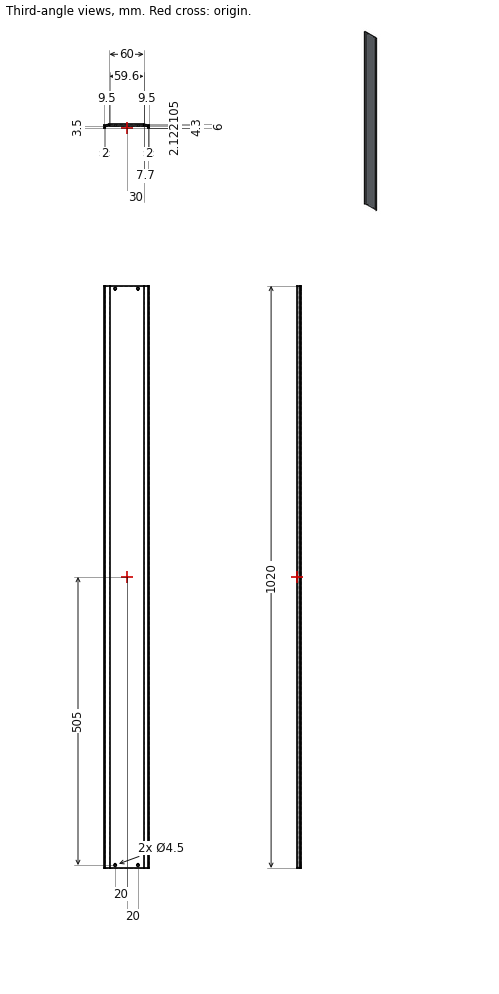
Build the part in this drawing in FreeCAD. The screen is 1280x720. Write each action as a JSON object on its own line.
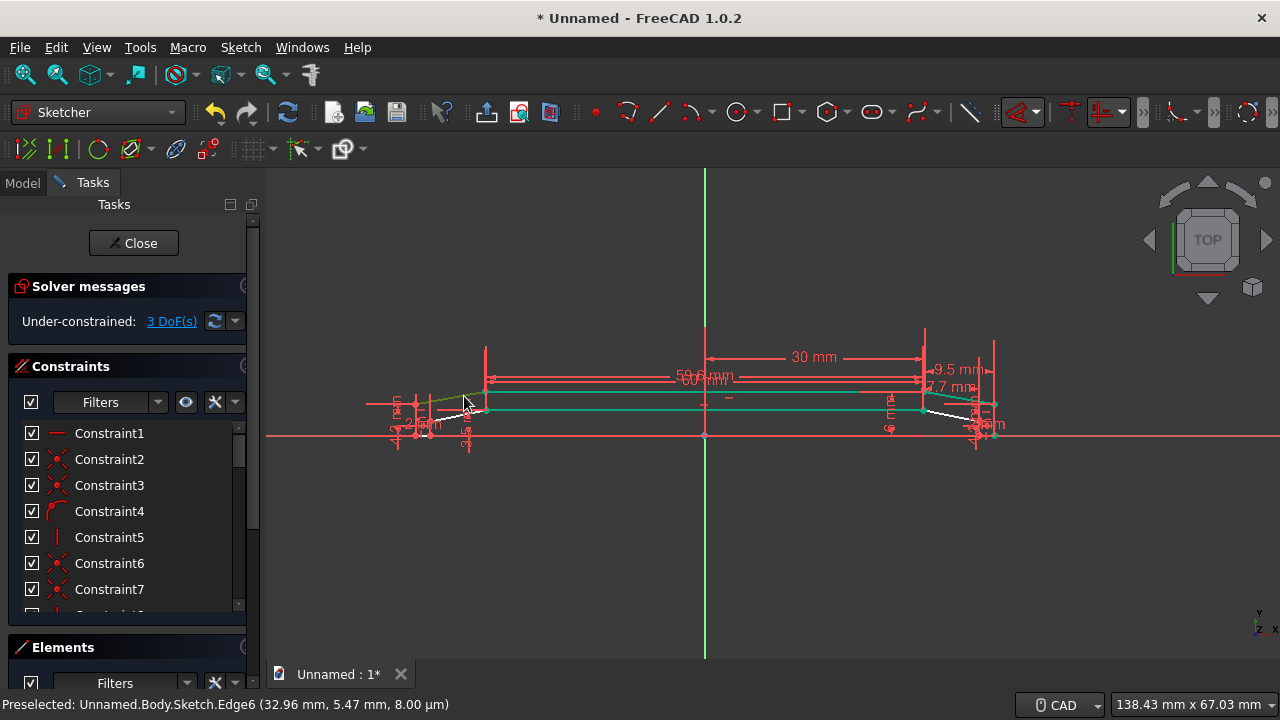
{"action": "key", "text": "l"}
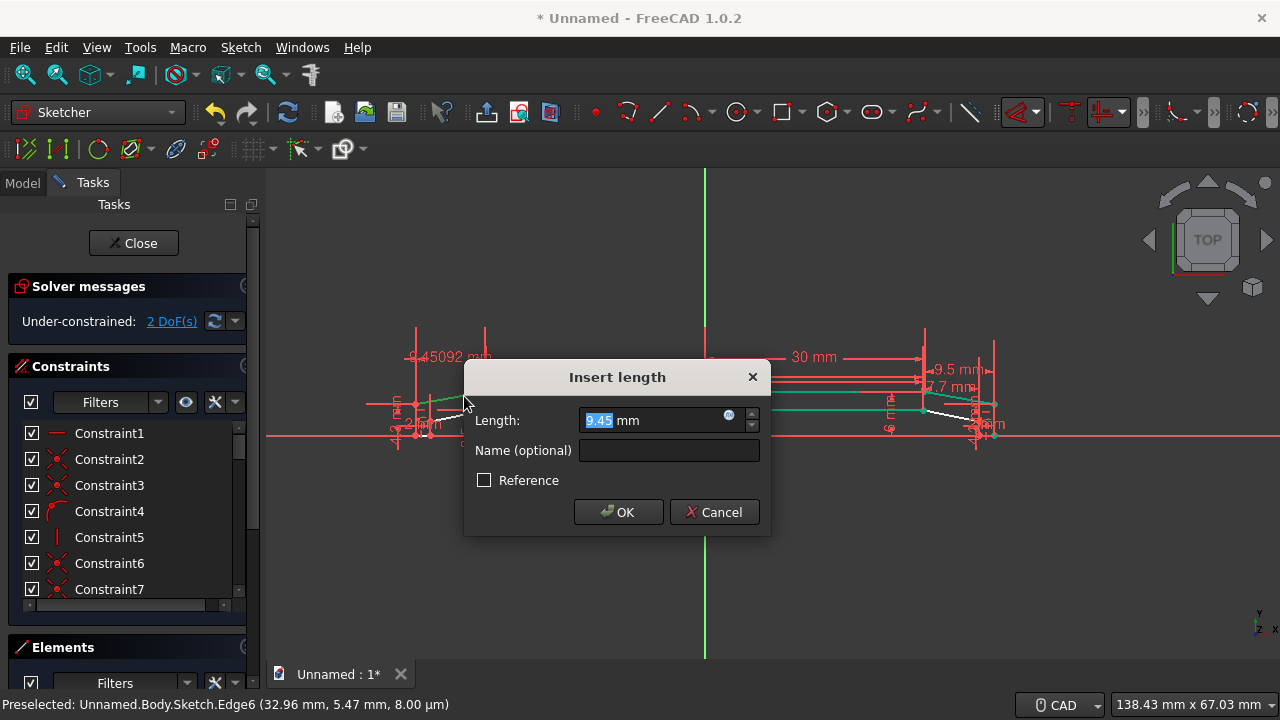
{"action": "type", "text": "9.5"}
{"action": "key", "text": "Return"}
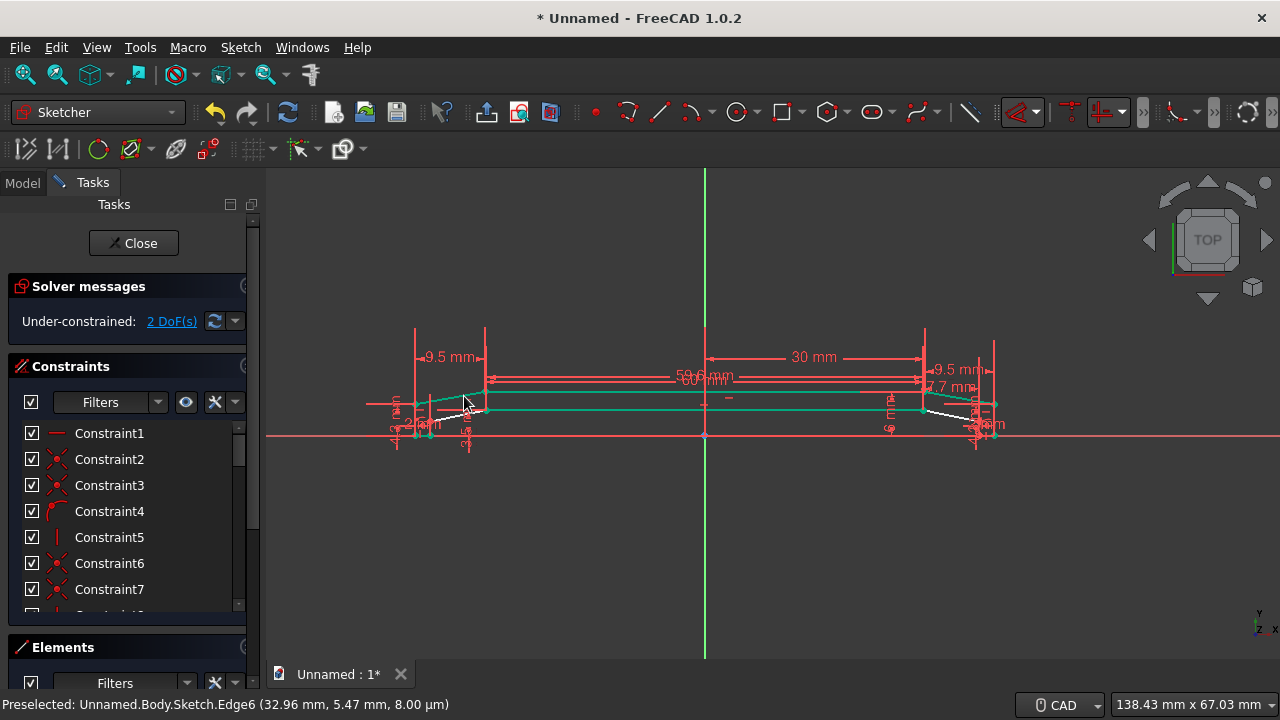
{"action": "scroll", "coordinate": [979, 429], "scroll_direction": "up", "scroll_amount": 5}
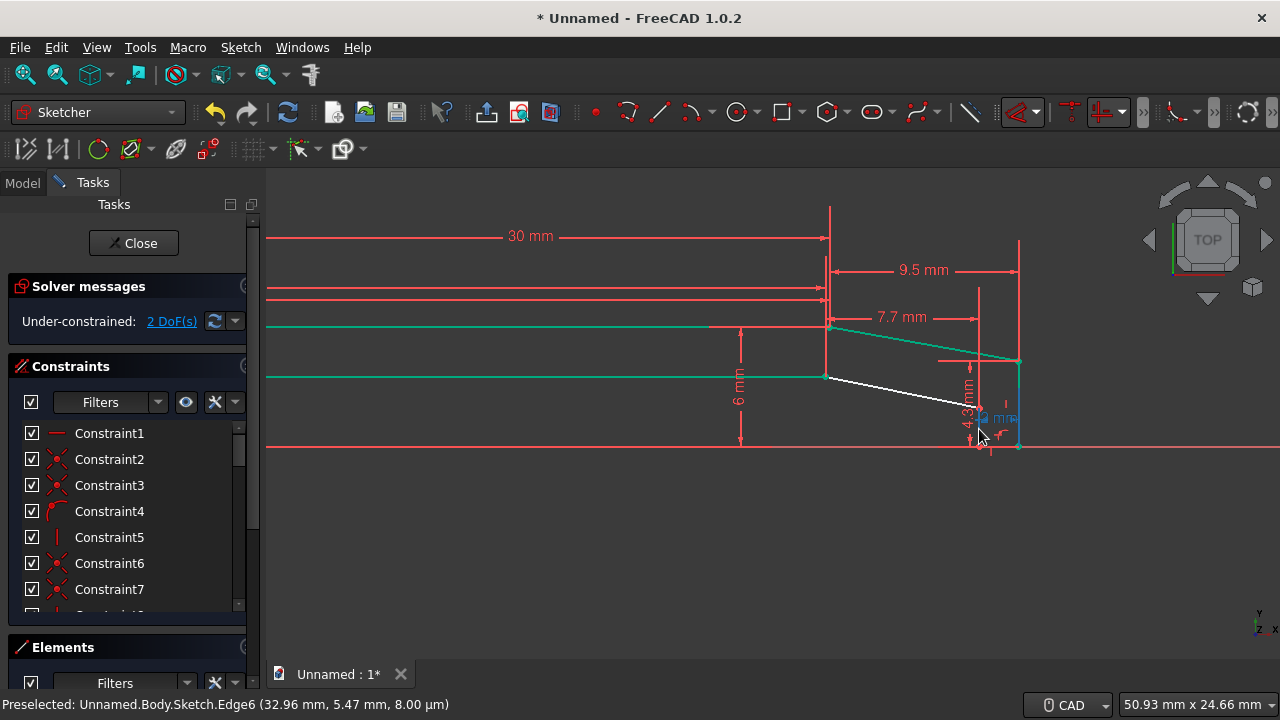
{"action": "left_click", "coordinate": [979, 427]}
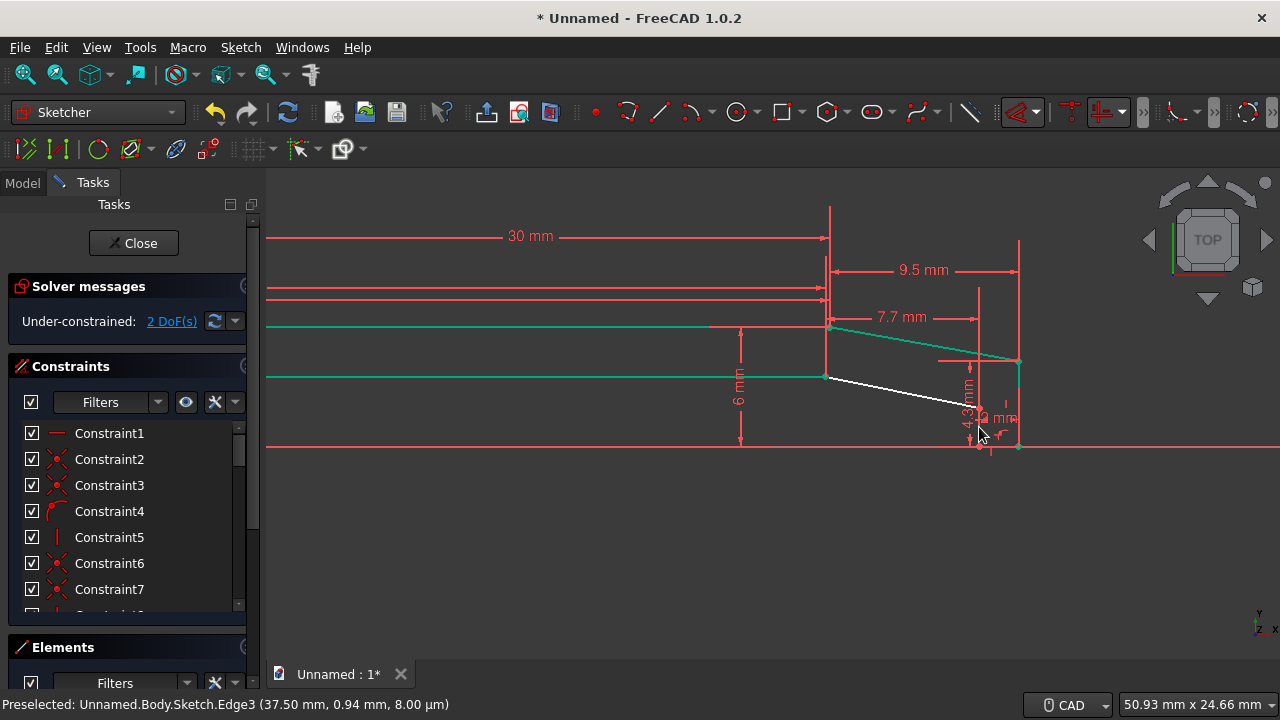
{"action": "key", "text": "i"}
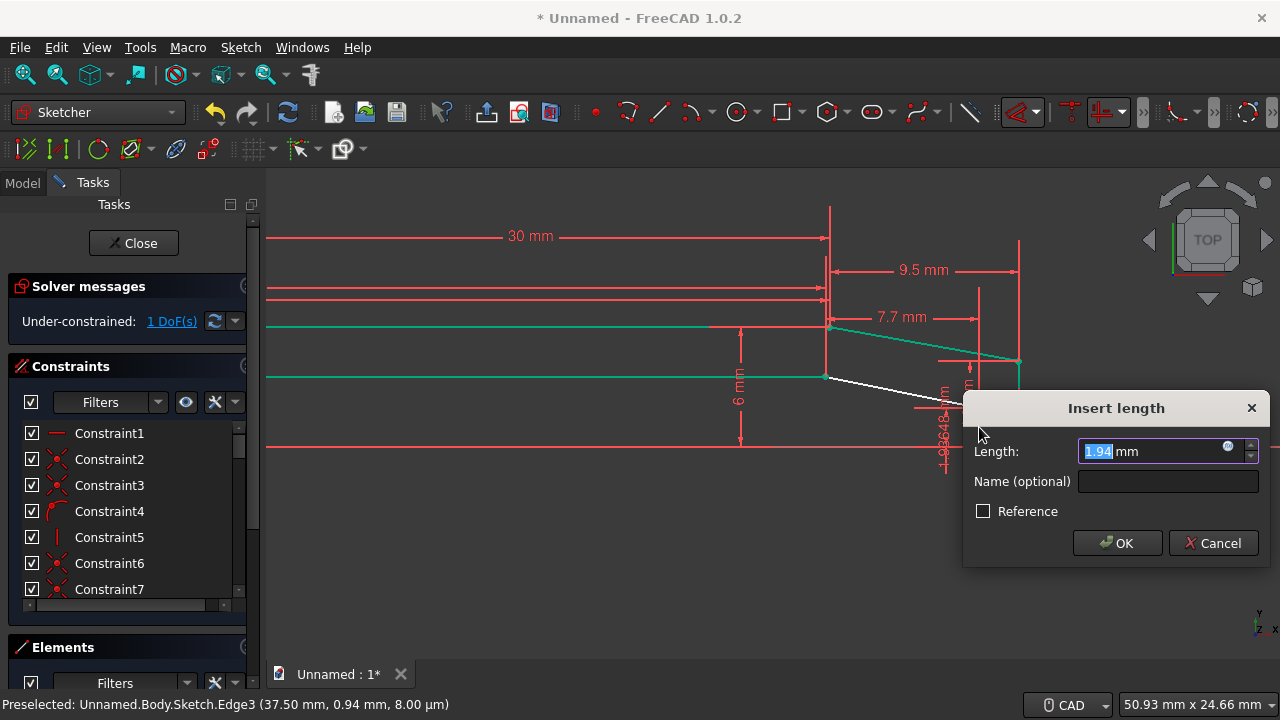
{"action": "type", "text": "2.122105"}
{"action": "key", "text": "Return"}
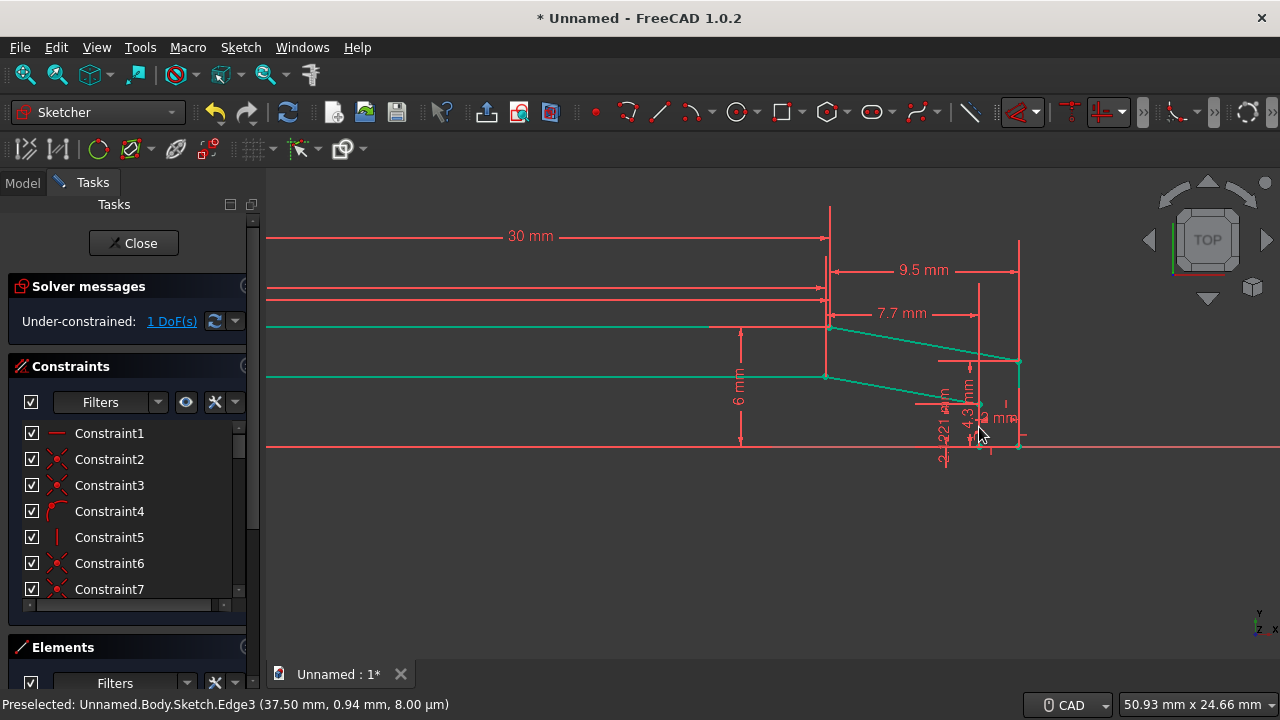
{"action": "scroll", "coordinate": [979, 429], "scroll_direction": "down", "scroll_amount": 5}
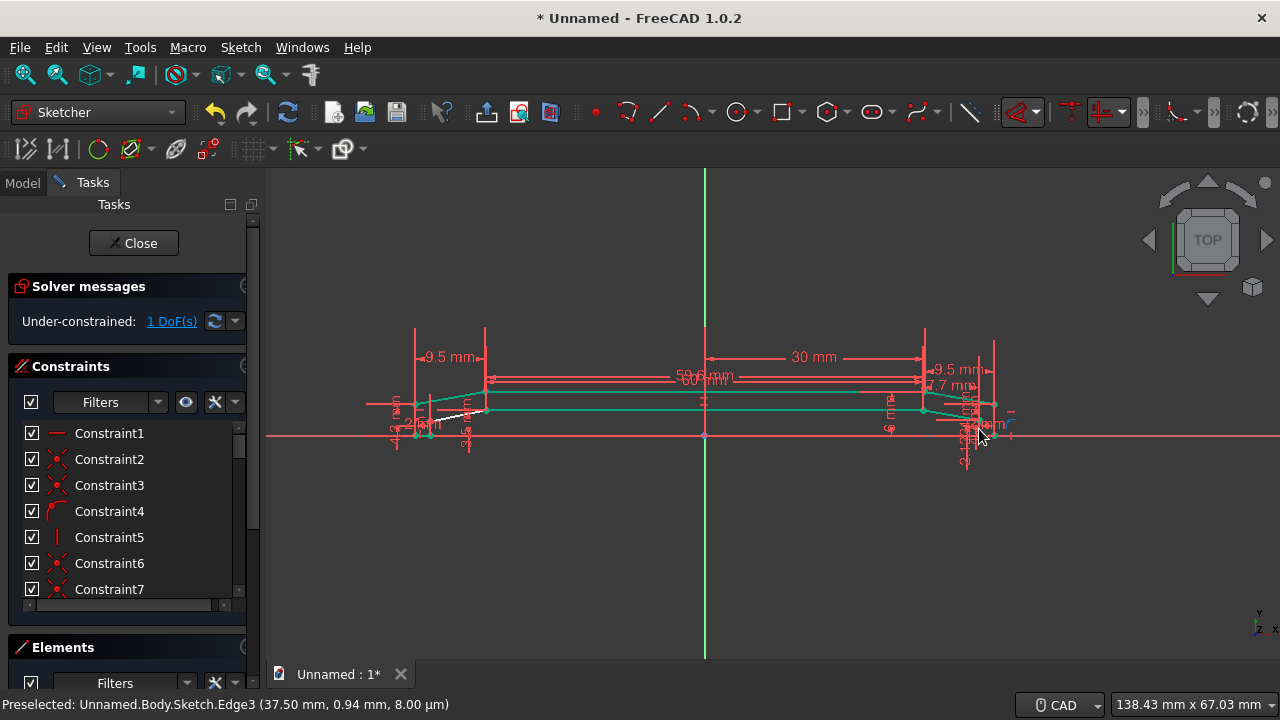
{"action": "scroll", "coordinate": [430, 432], "scroll_direction": "up", "scroll_amount": 6}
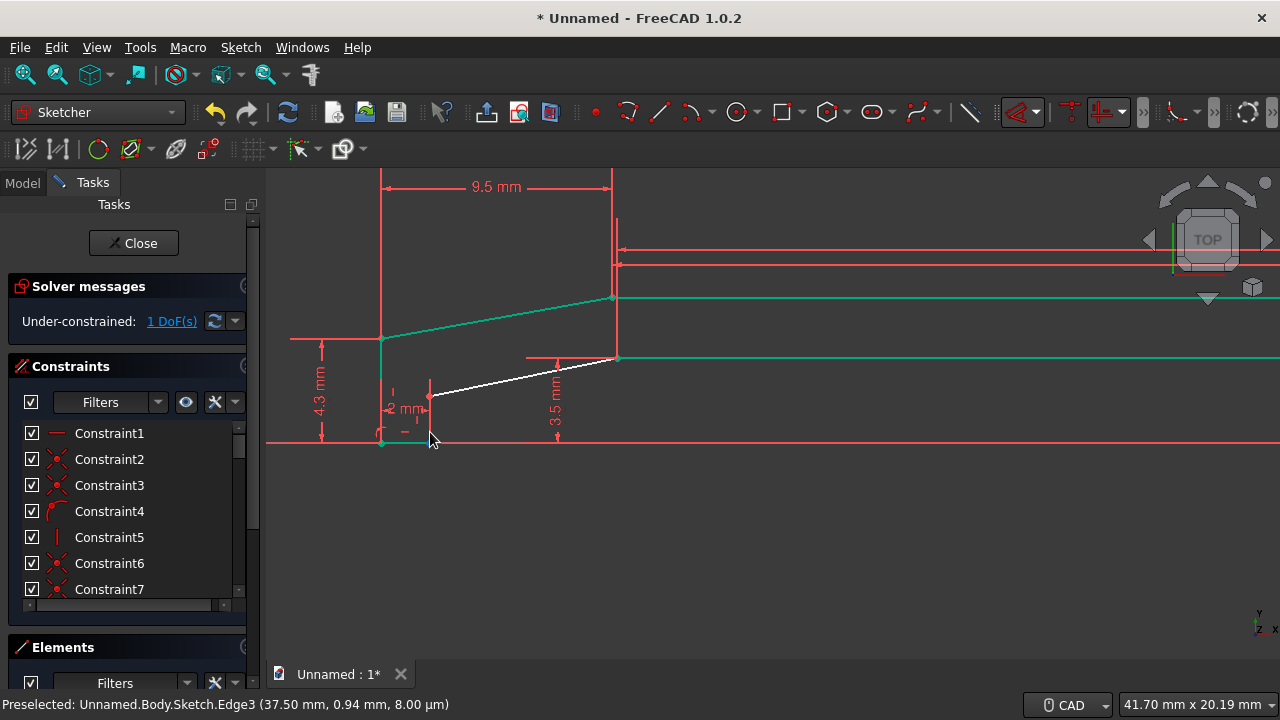
{"action": "left_click", "coordinate": [430, 429]}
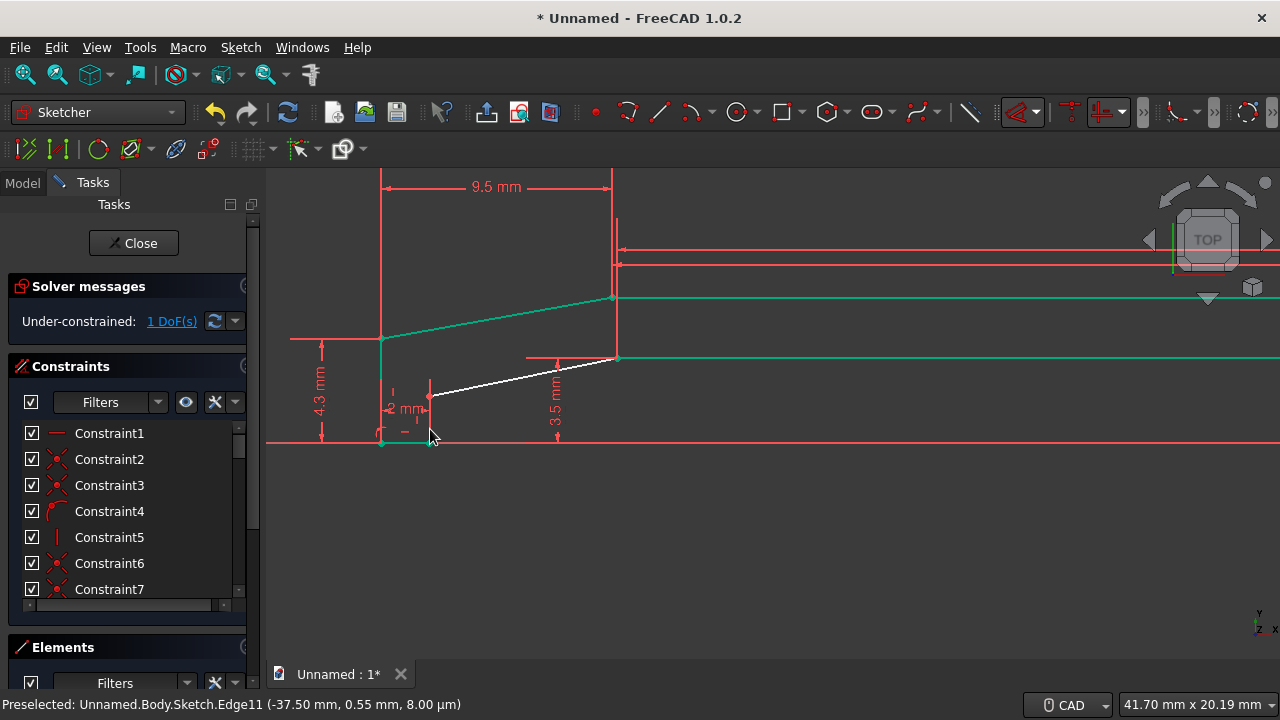
{"action": "key", "text": "i"}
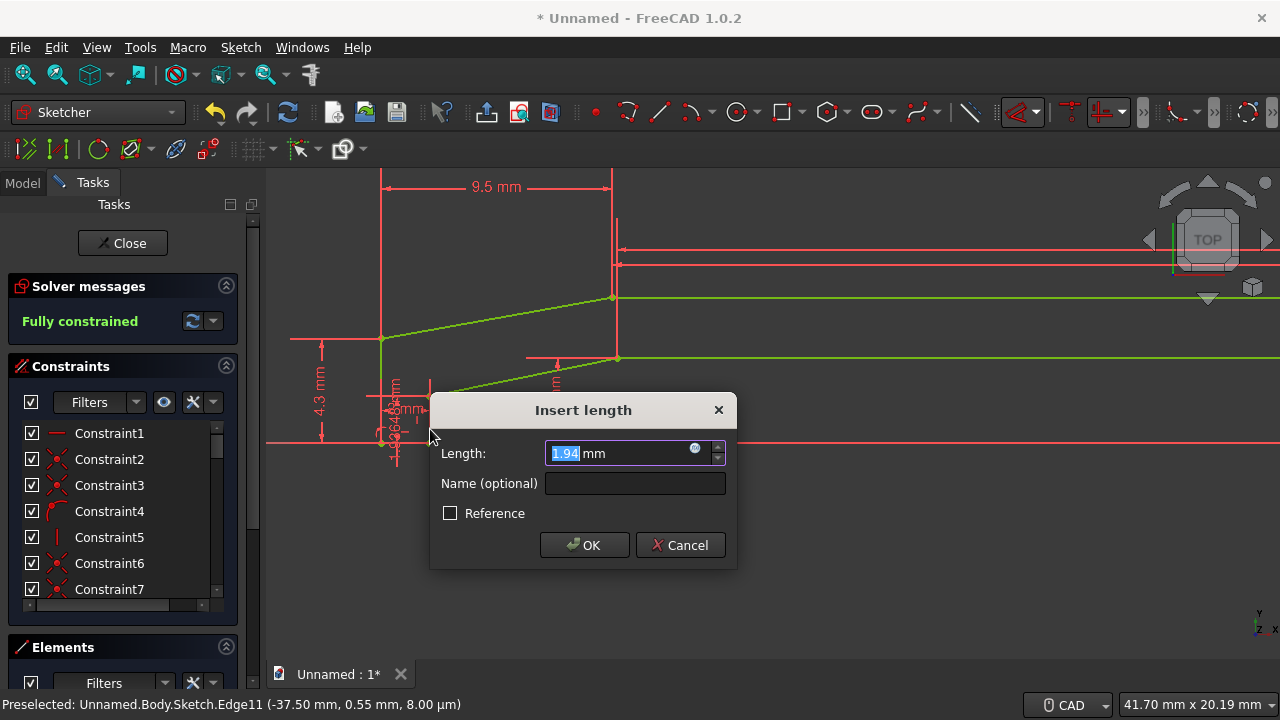
{"action": "type", "text": "2.122105"}
{"action": "key", "text": "Return"}